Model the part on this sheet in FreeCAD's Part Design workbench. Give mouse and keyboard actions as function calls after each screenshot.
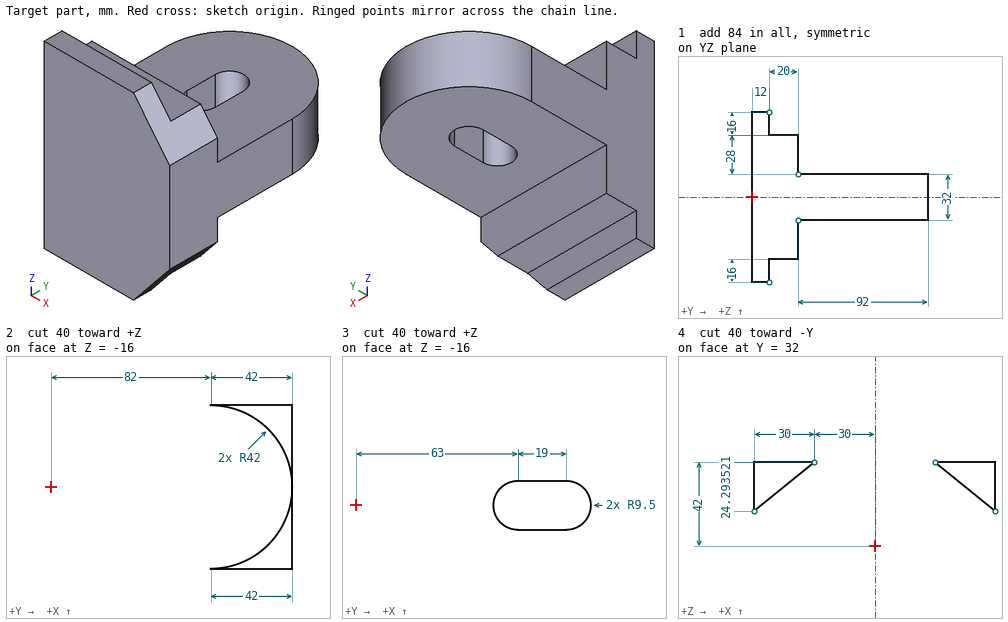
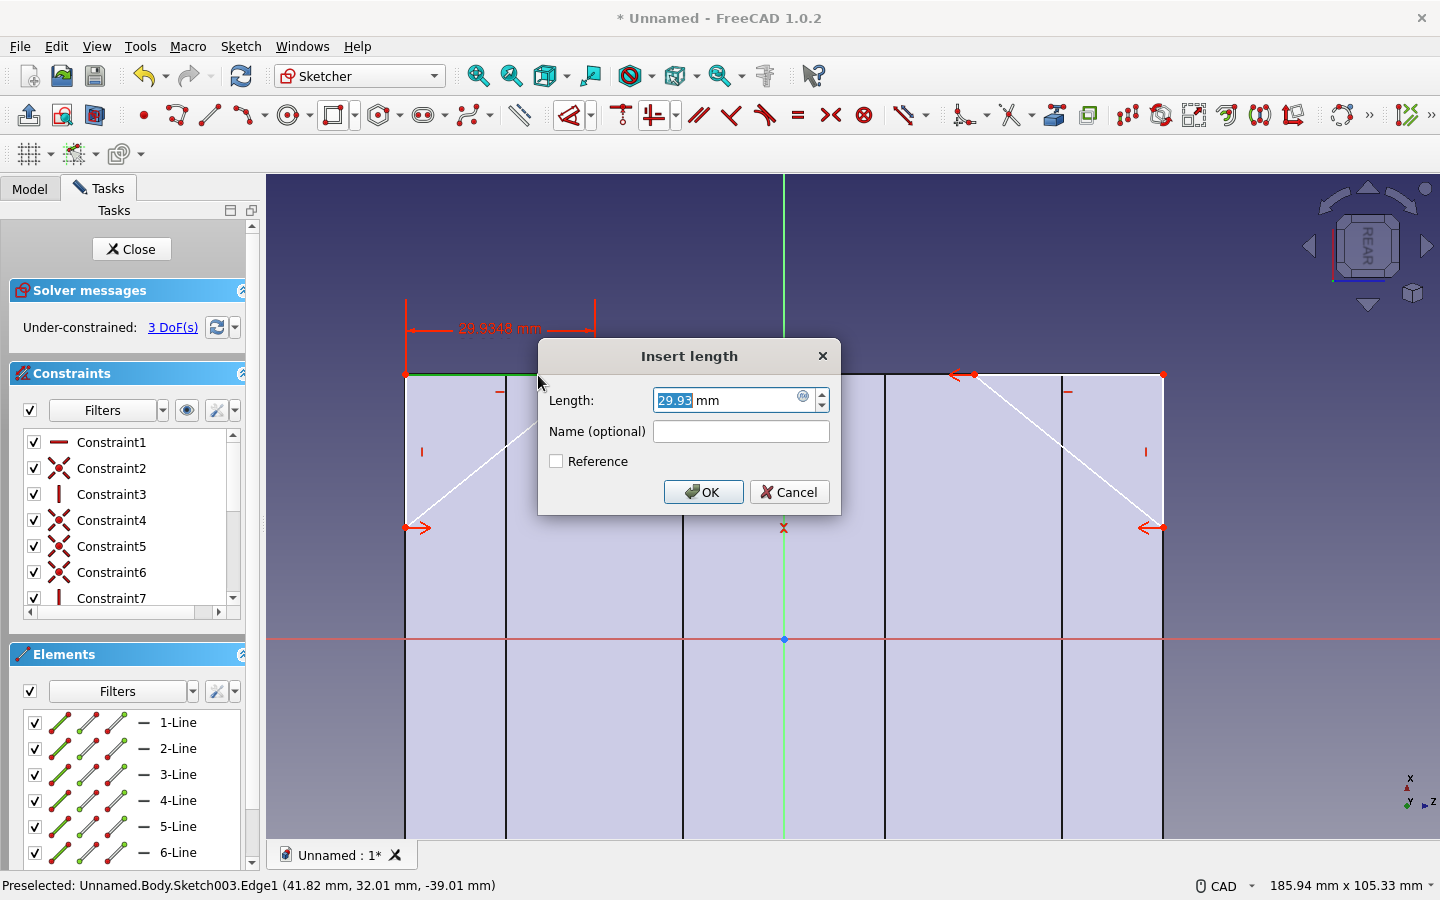
text(30)
key(Return)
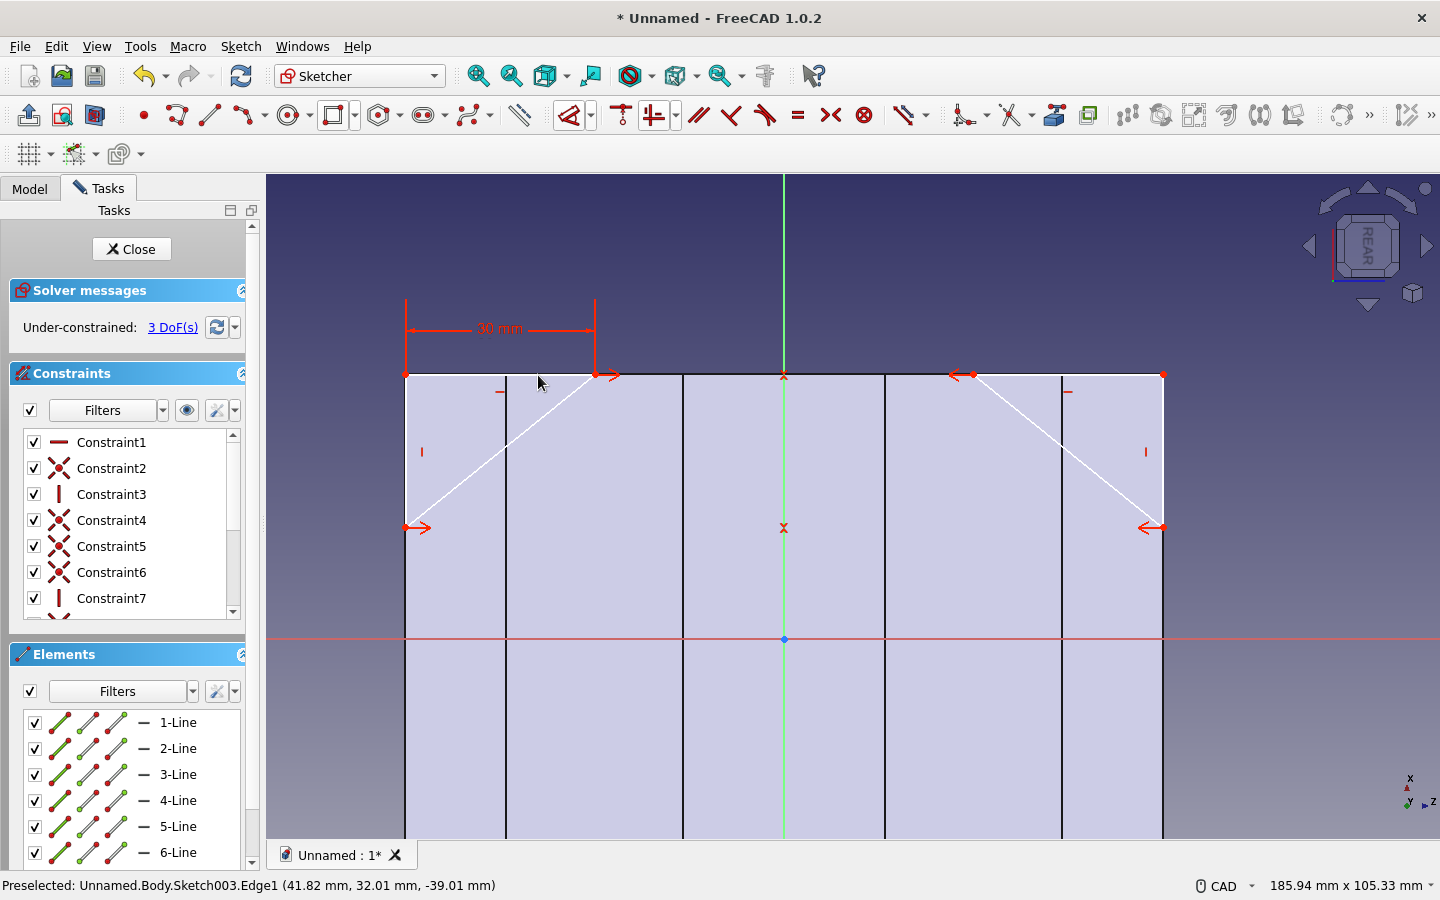
click(595, 375)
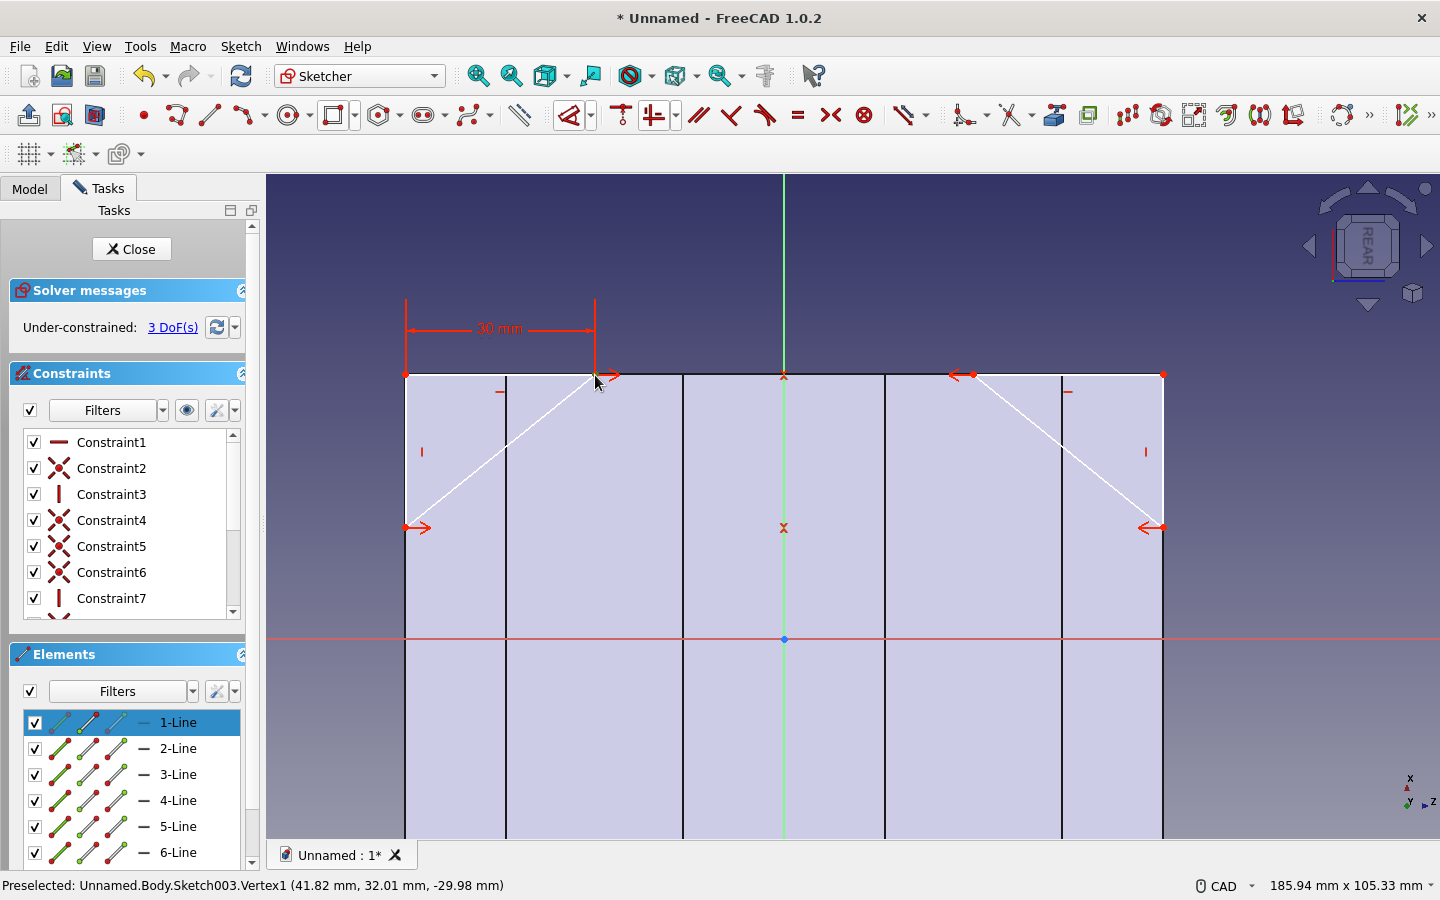
key(l)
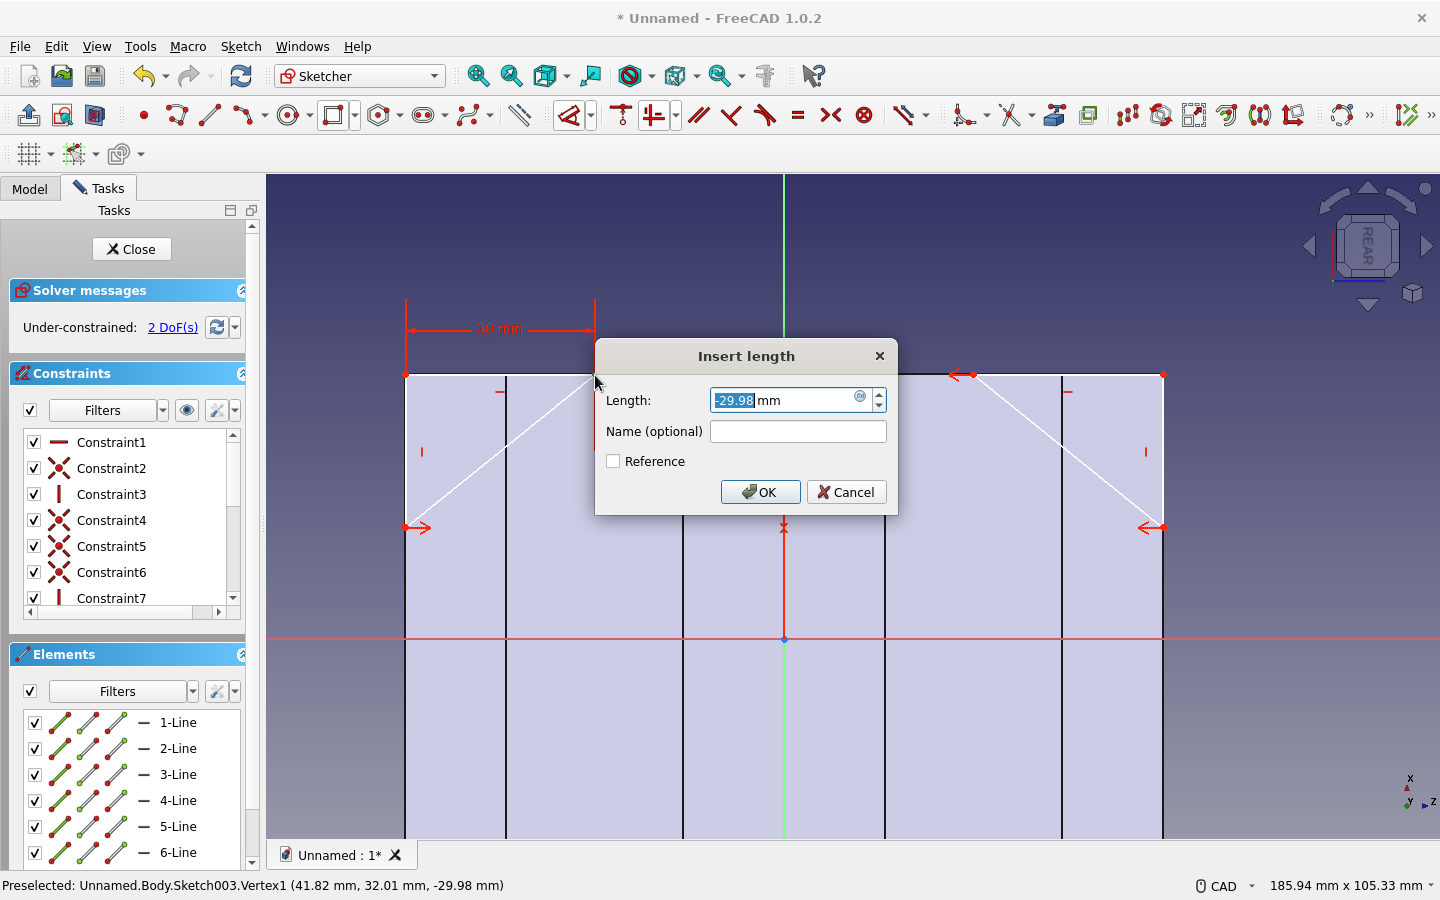
text(-30)
key(Return)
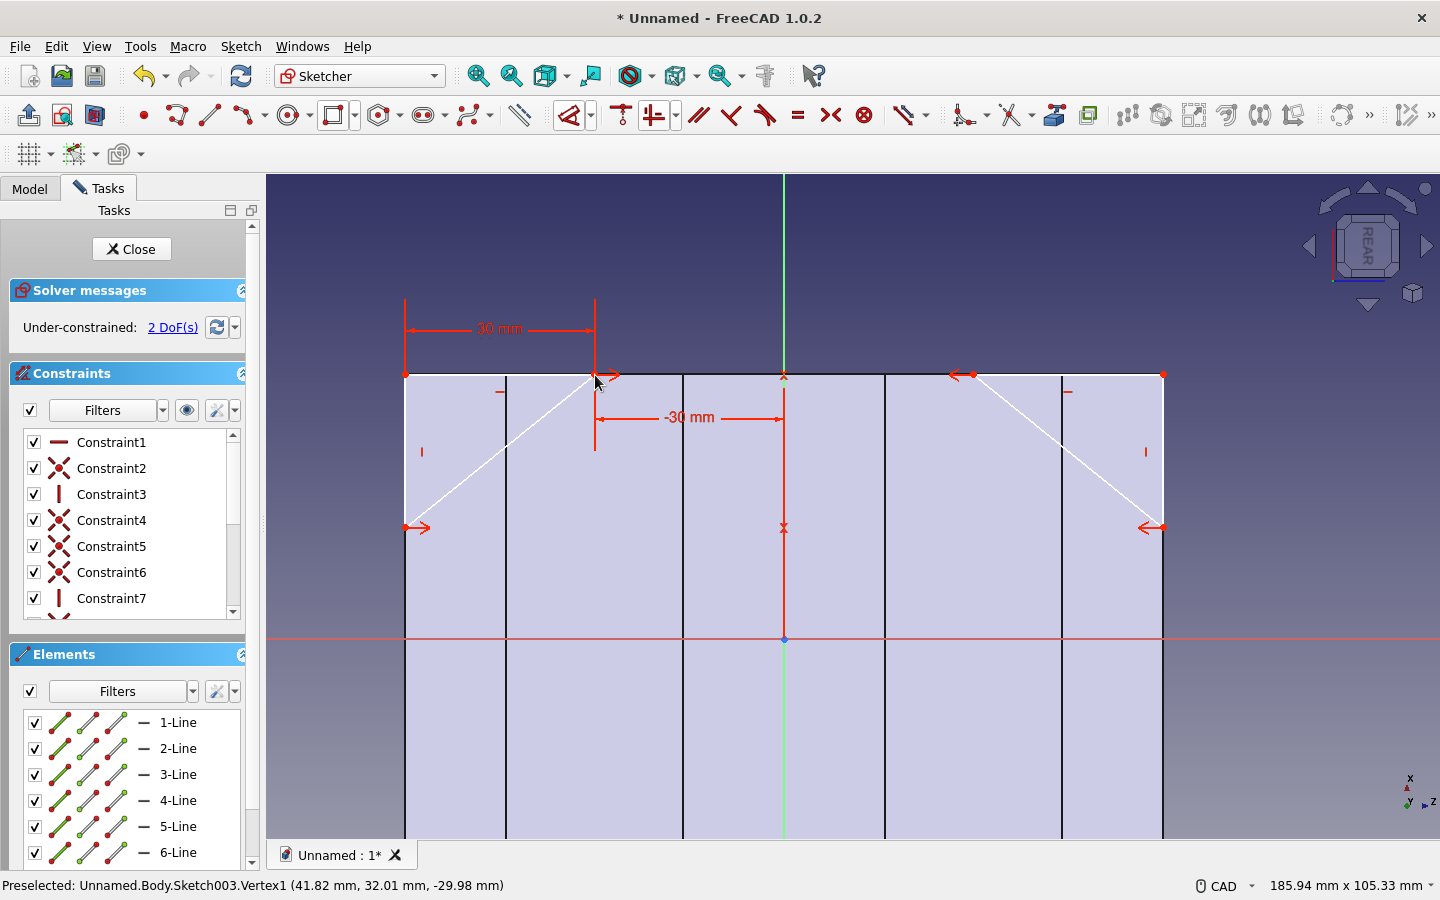
click(595, 375)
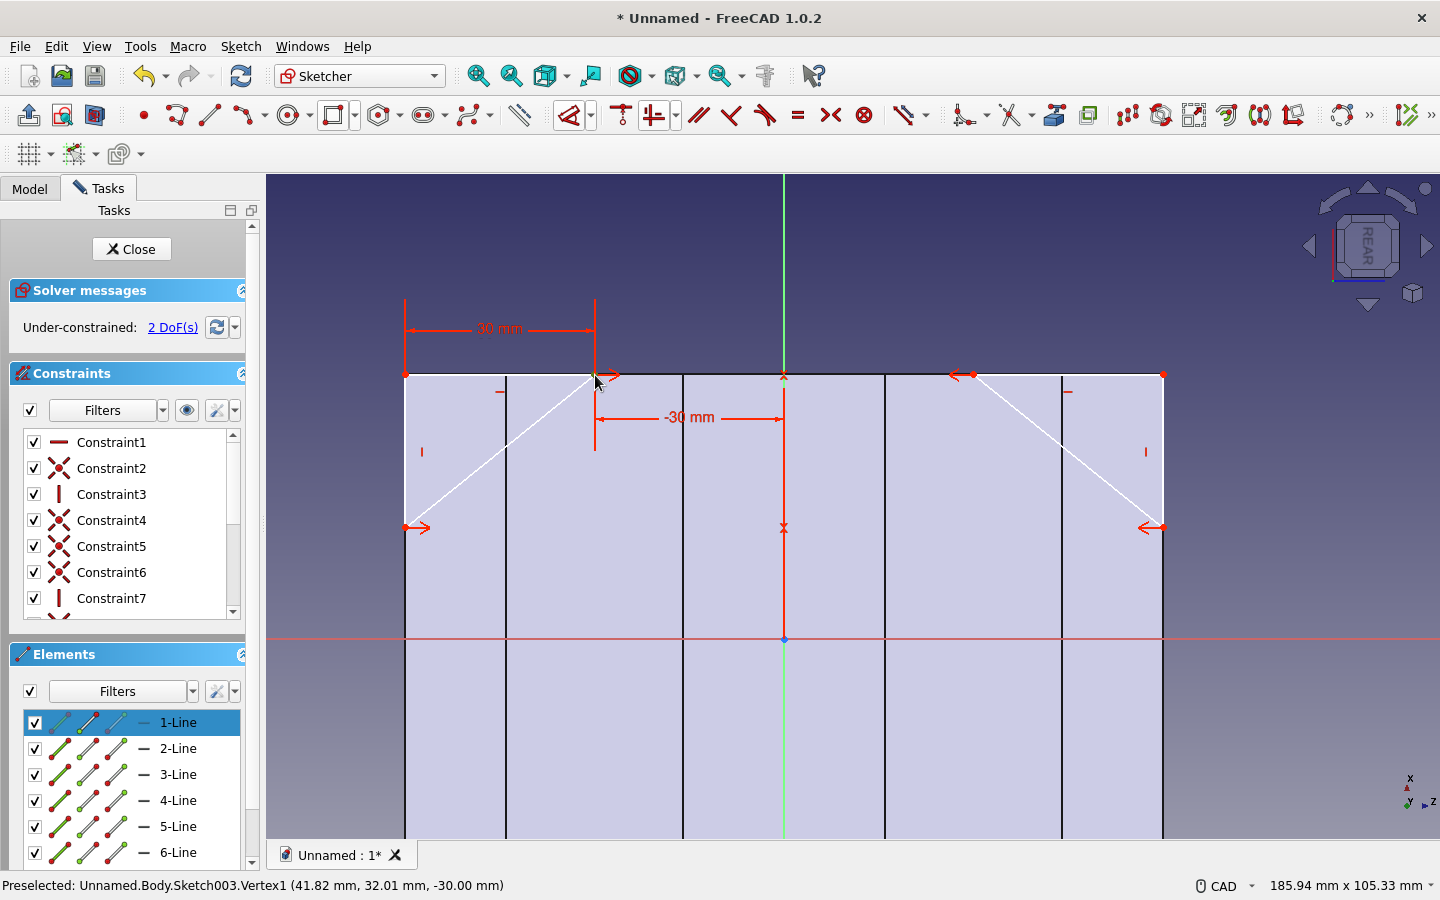
click(590, 116)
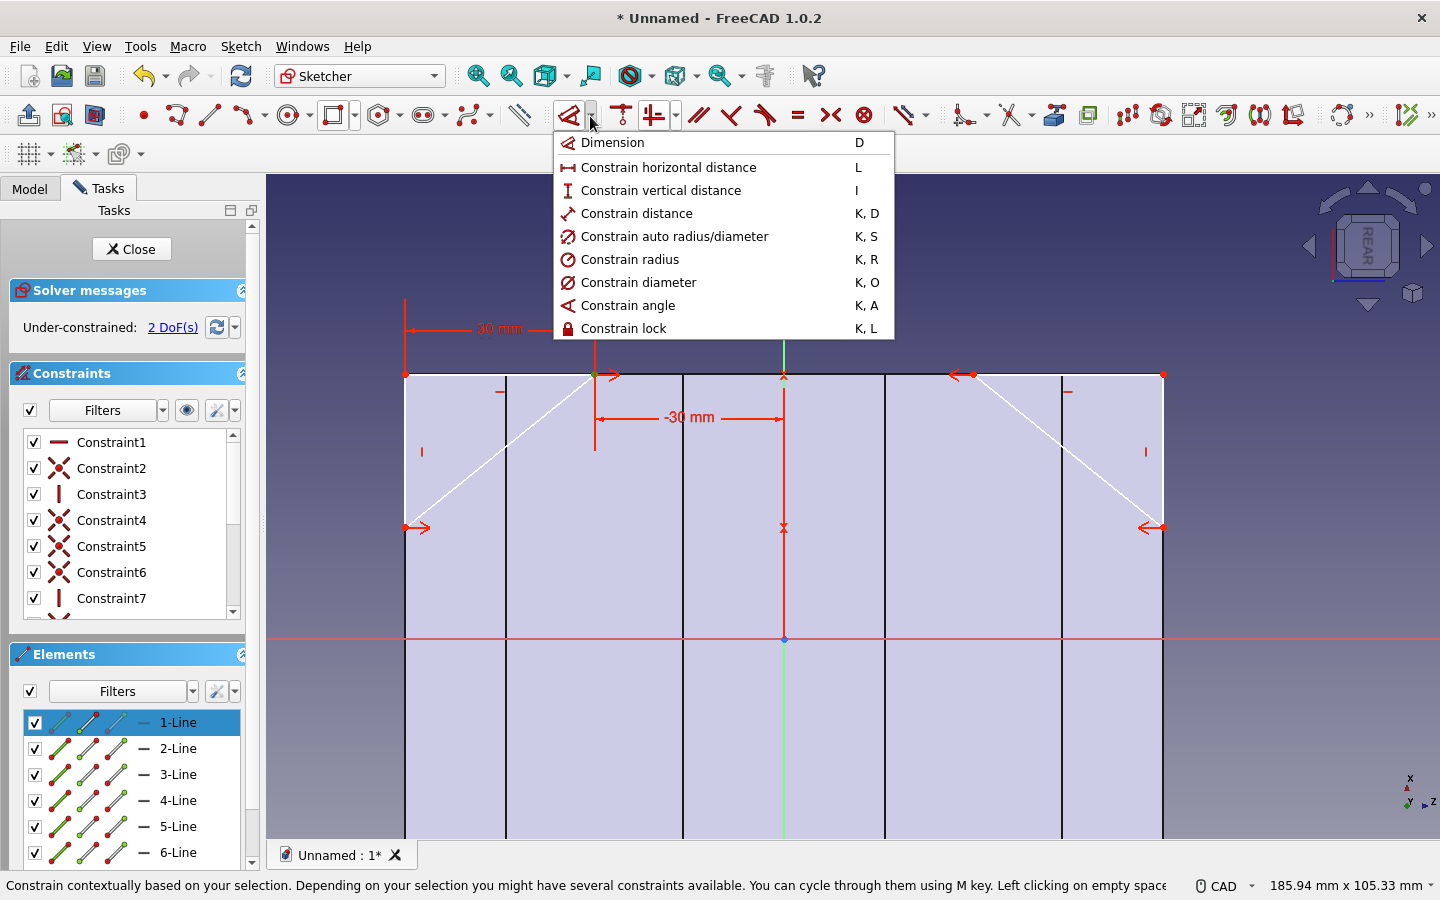
click(724, 190)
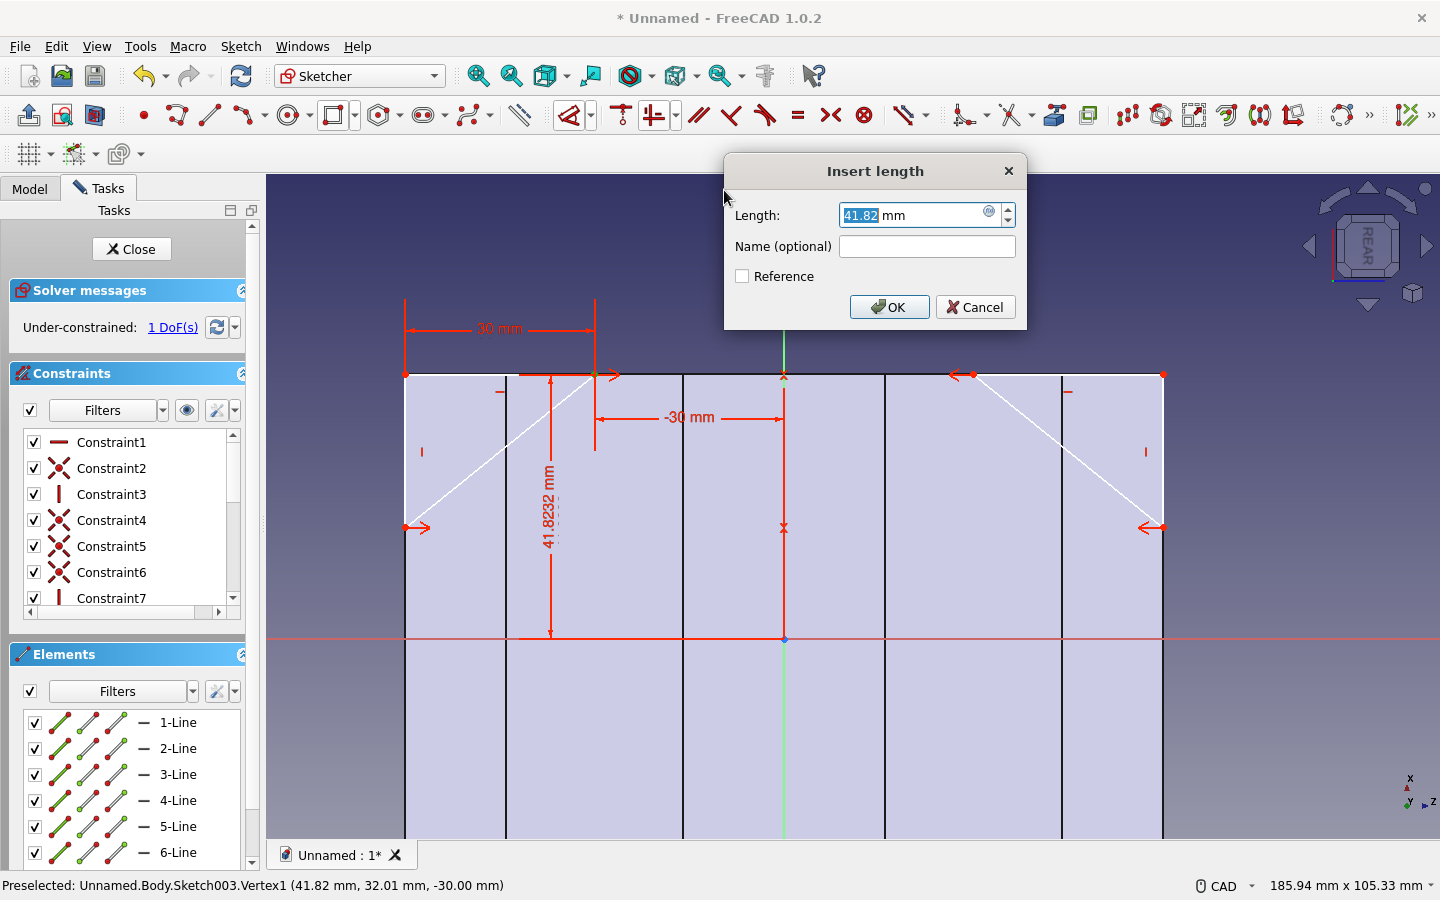
text(42)
key(Return)